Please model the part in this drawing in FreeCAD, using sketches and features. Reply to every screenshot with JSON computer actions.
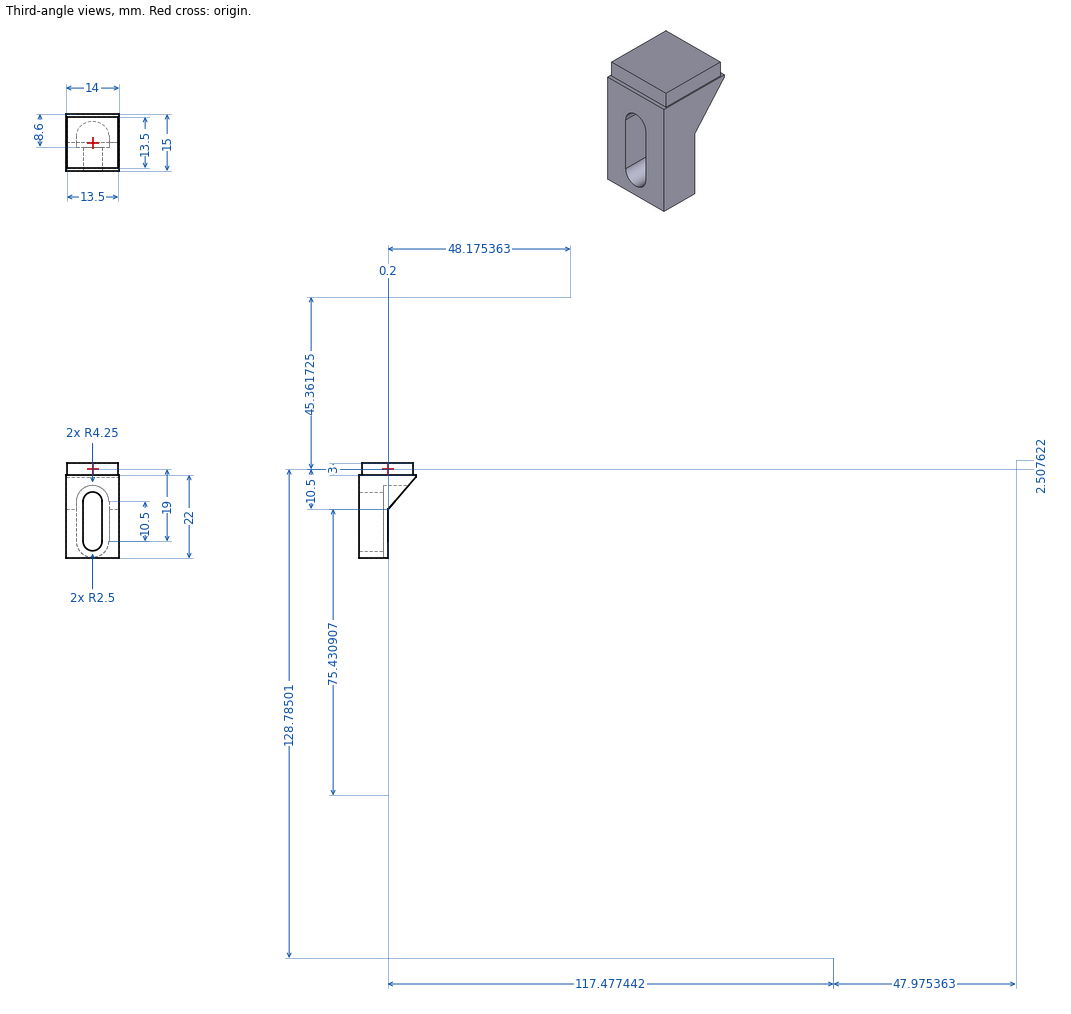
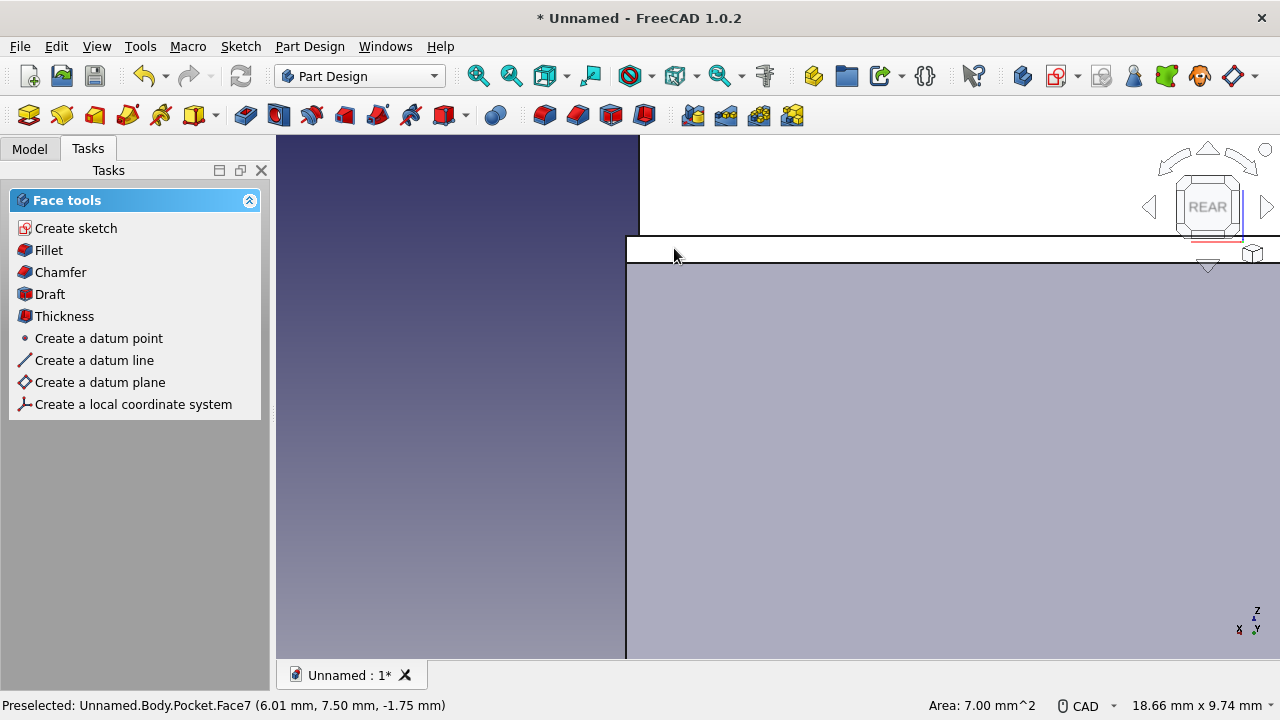
{"action": "left_click", "coordinate": [1056, 76]}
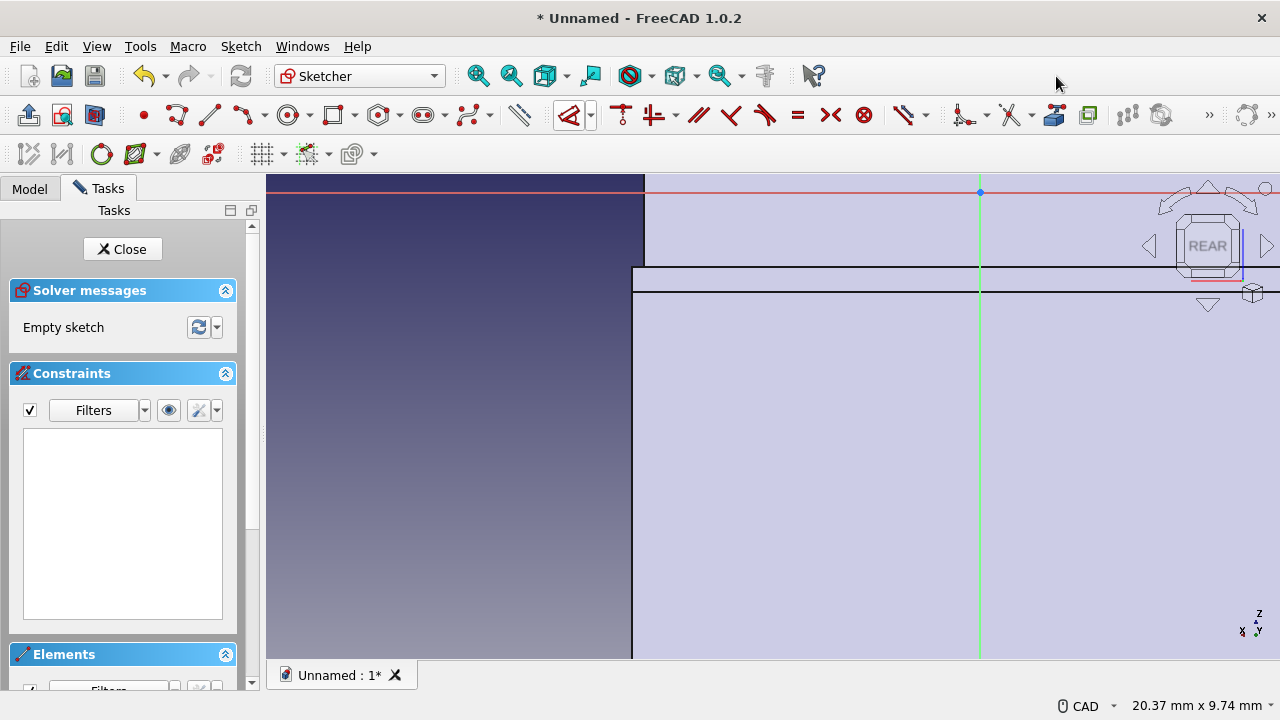
{"action": "scroll", "coordinate": [614, 300], "scroll_direction": "down", "scroll_amount": 7}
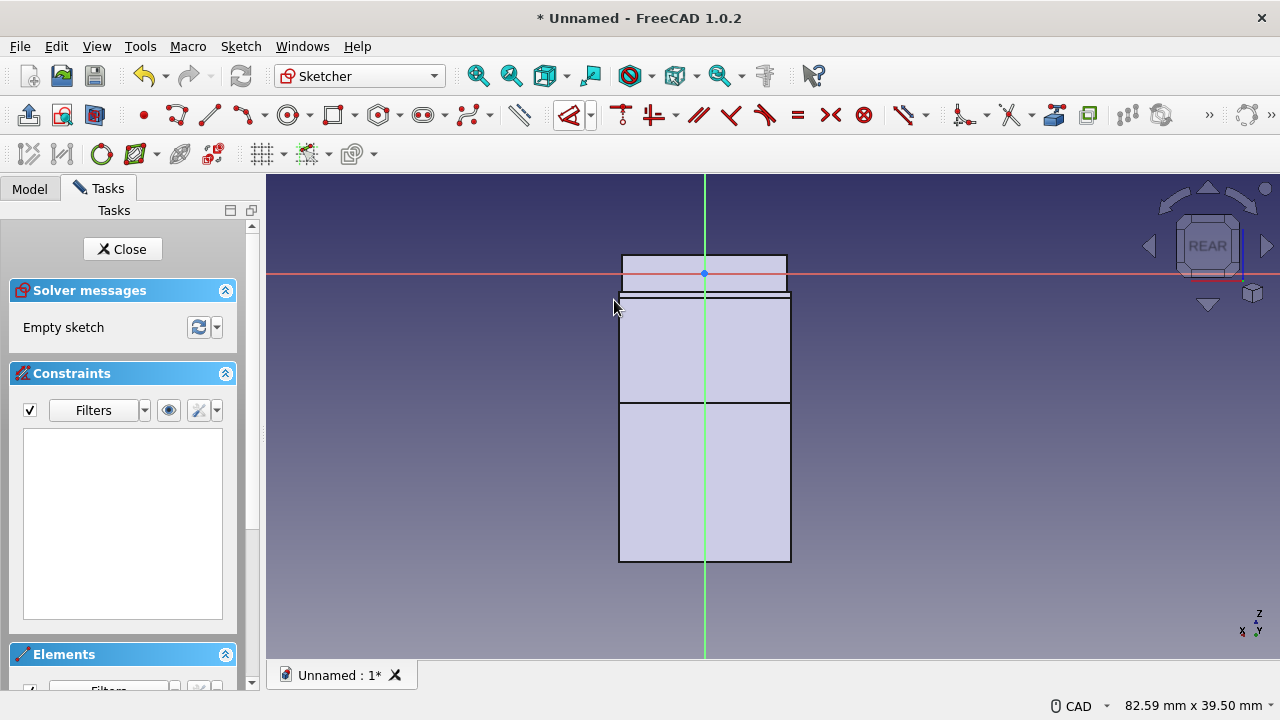
{"action": "key", "text": "g s"}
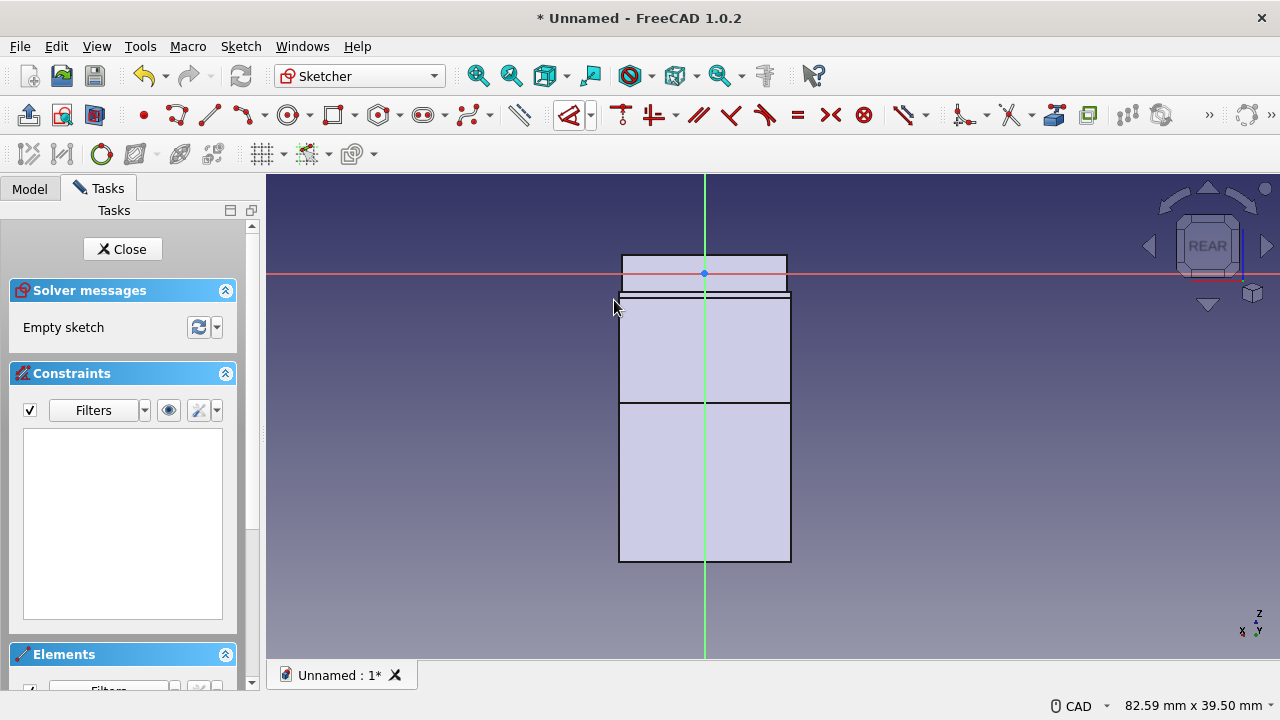
{"action": "left_click", "coordinate": [705, 507]}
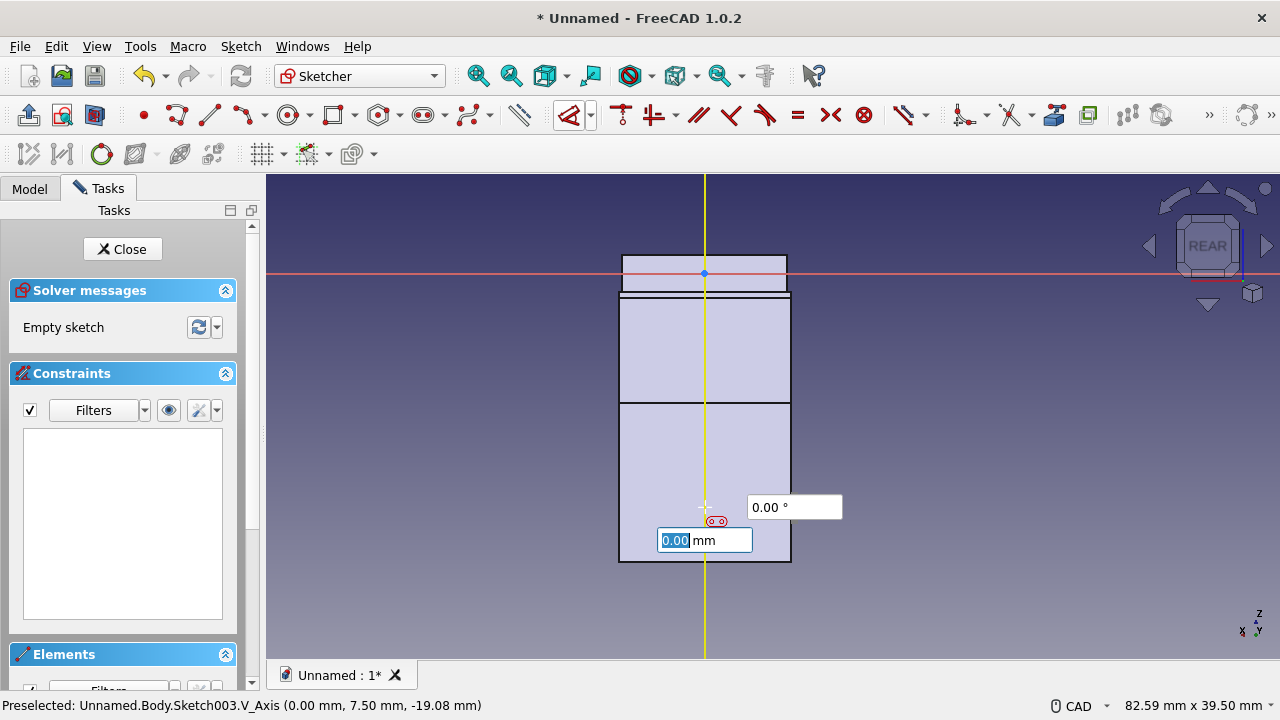
{"action": "left_click", "coordinate": [714, 378]}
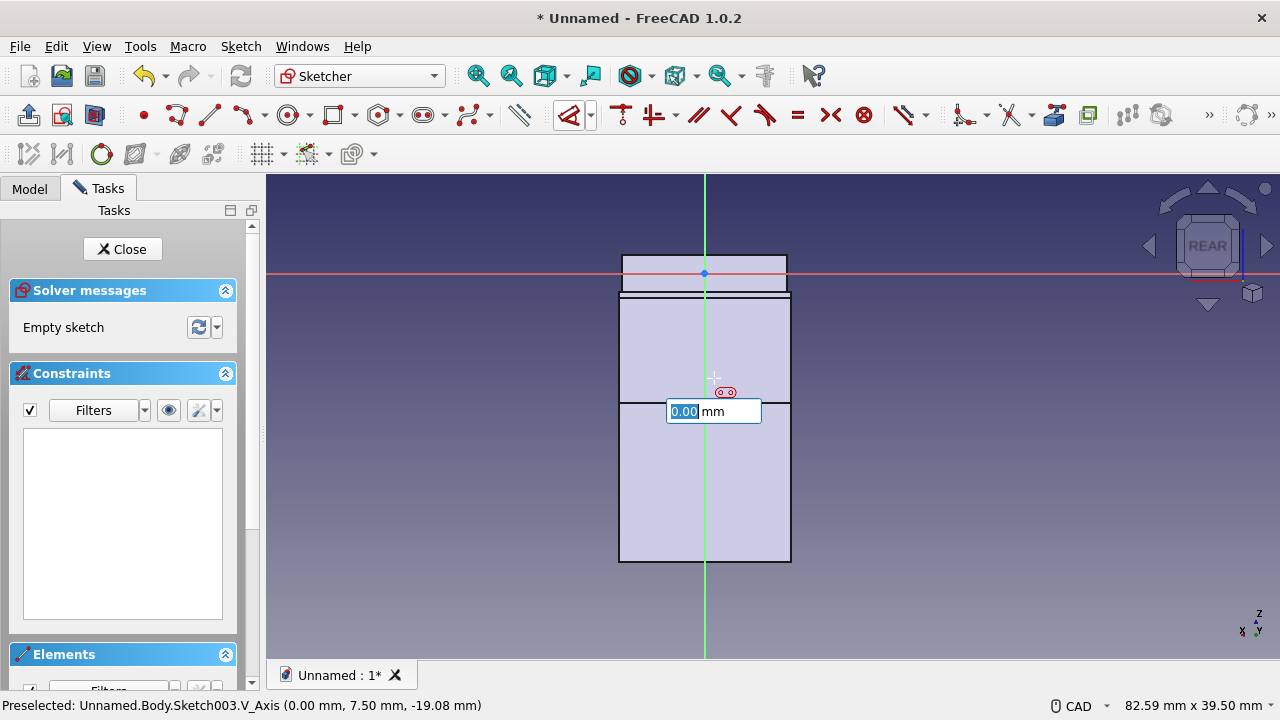
{"action": "left_click", "coordinate": [757, 443]}
{"action": "key", "text": "Escape"}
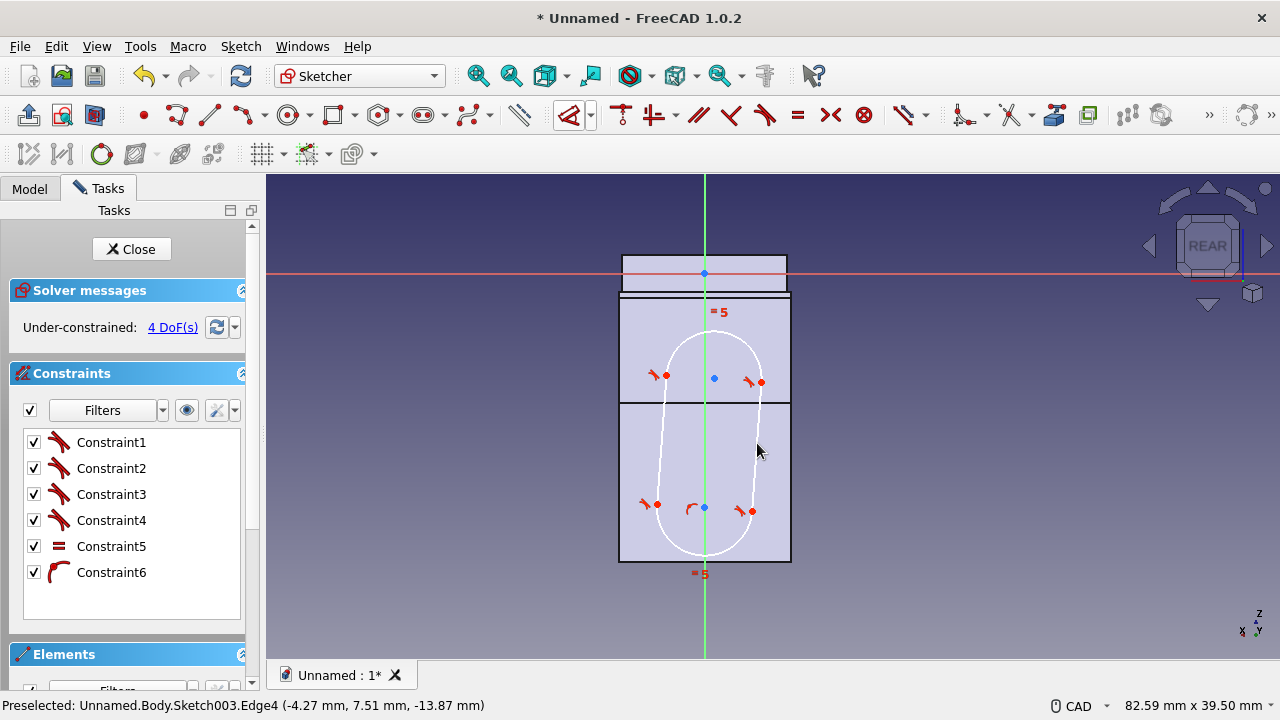
{"action": "left_click", "coordinate": [660, 466]}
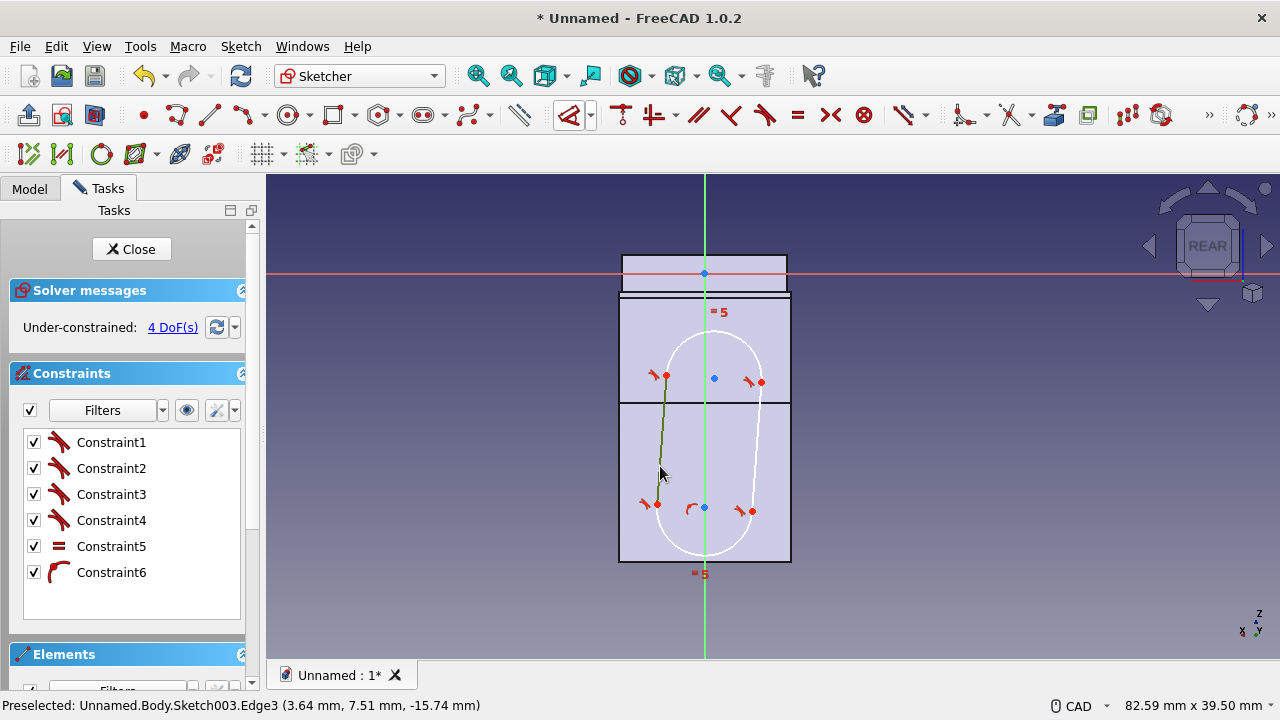
{"action": "key", "text": "v"}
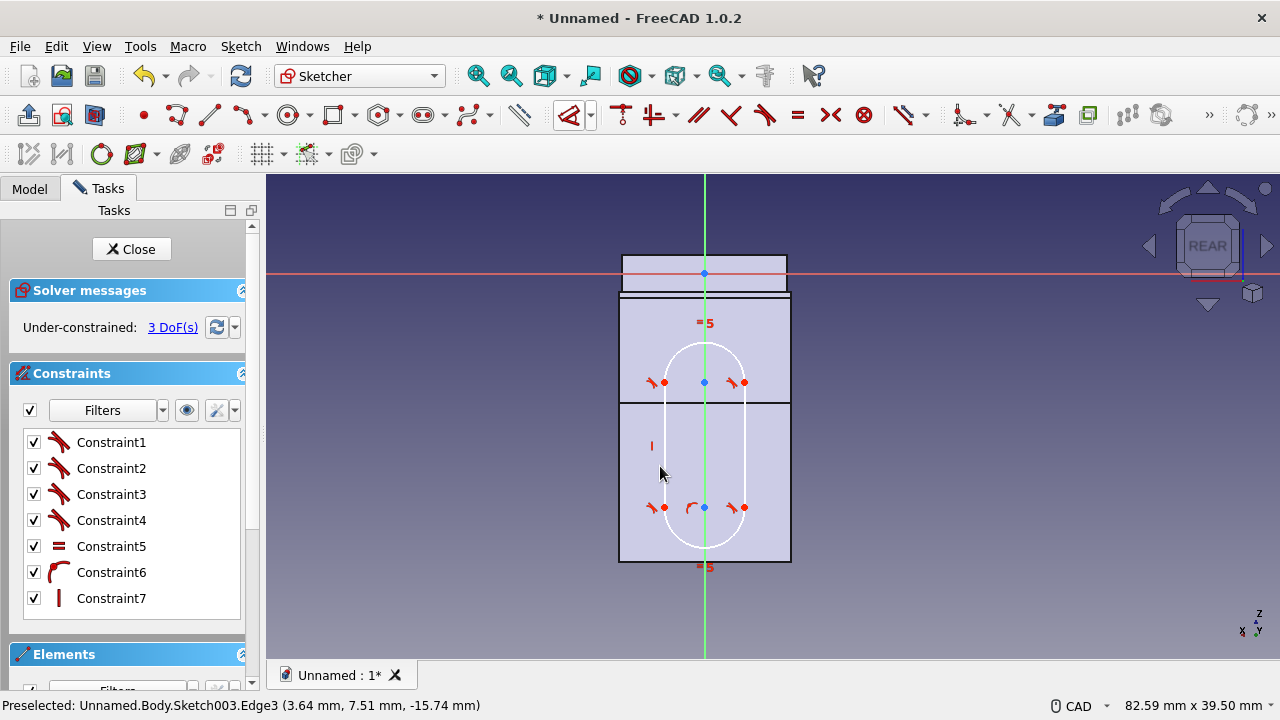
{"action": "left_click", "coordinate": [681, 540]}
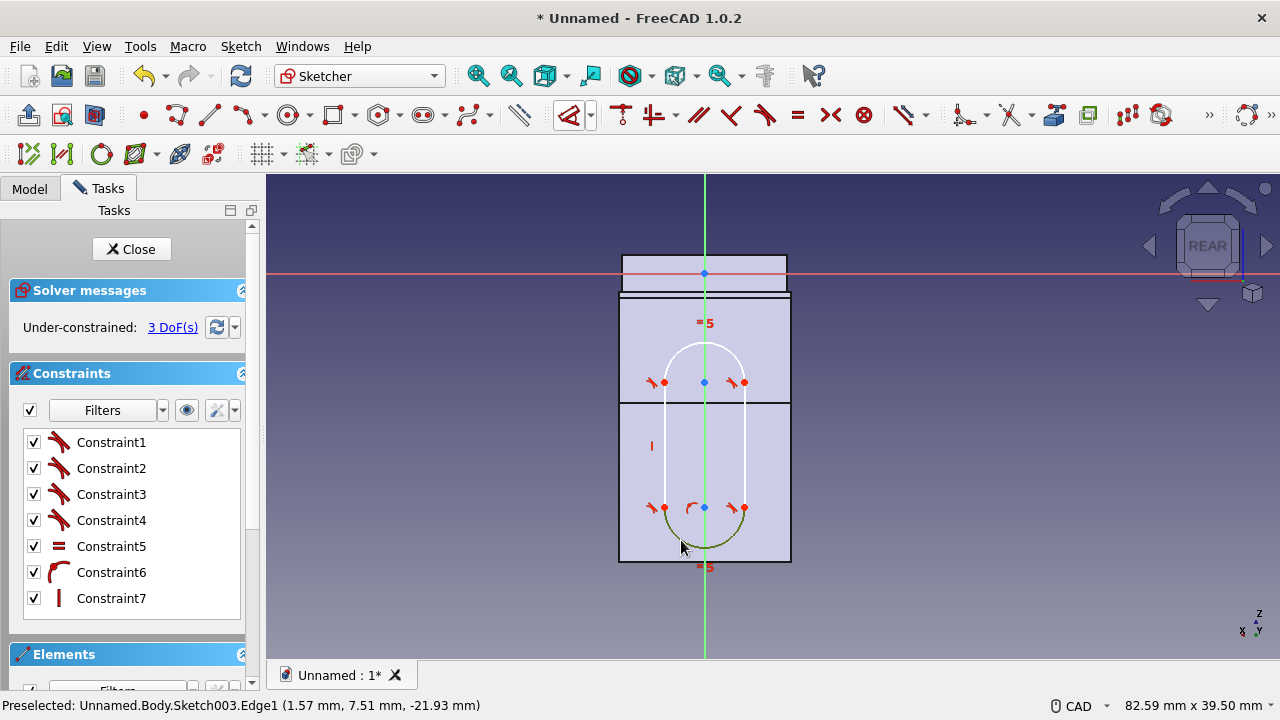
{"action": "key", "text": "k r"}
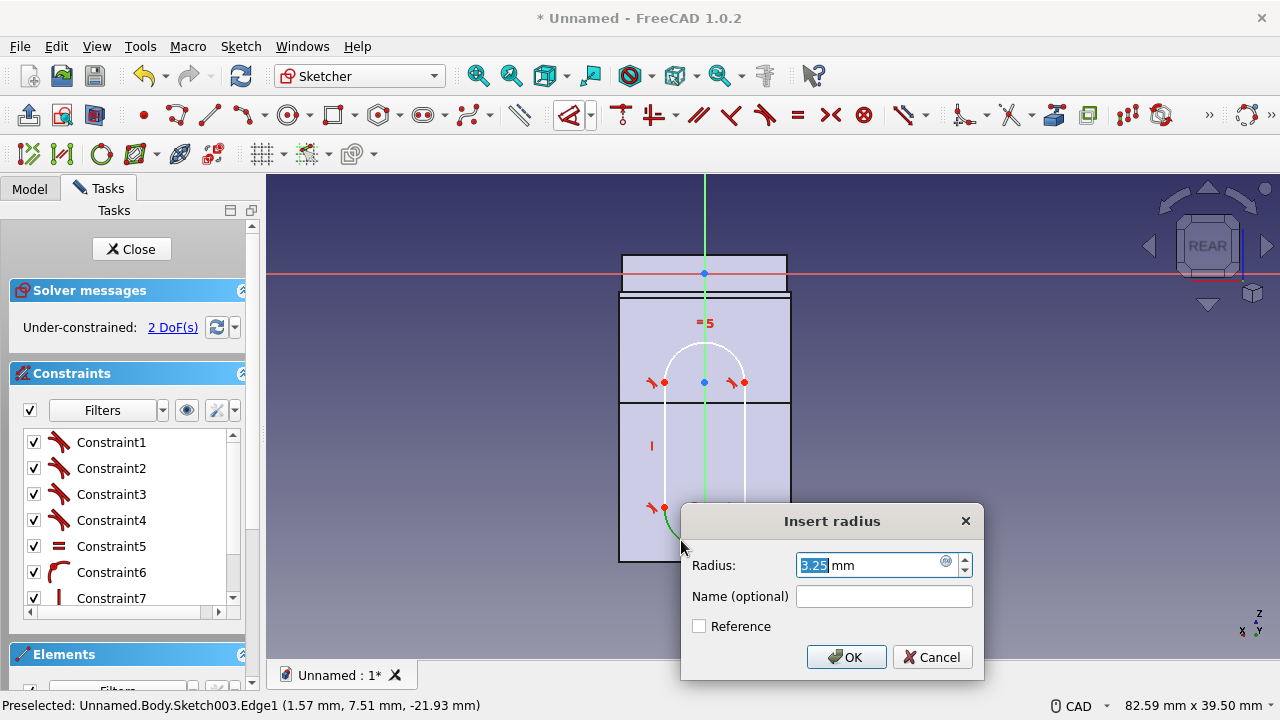
{"action": "type", "text": "4.25"}
{"action": "key", "text": "Return"}